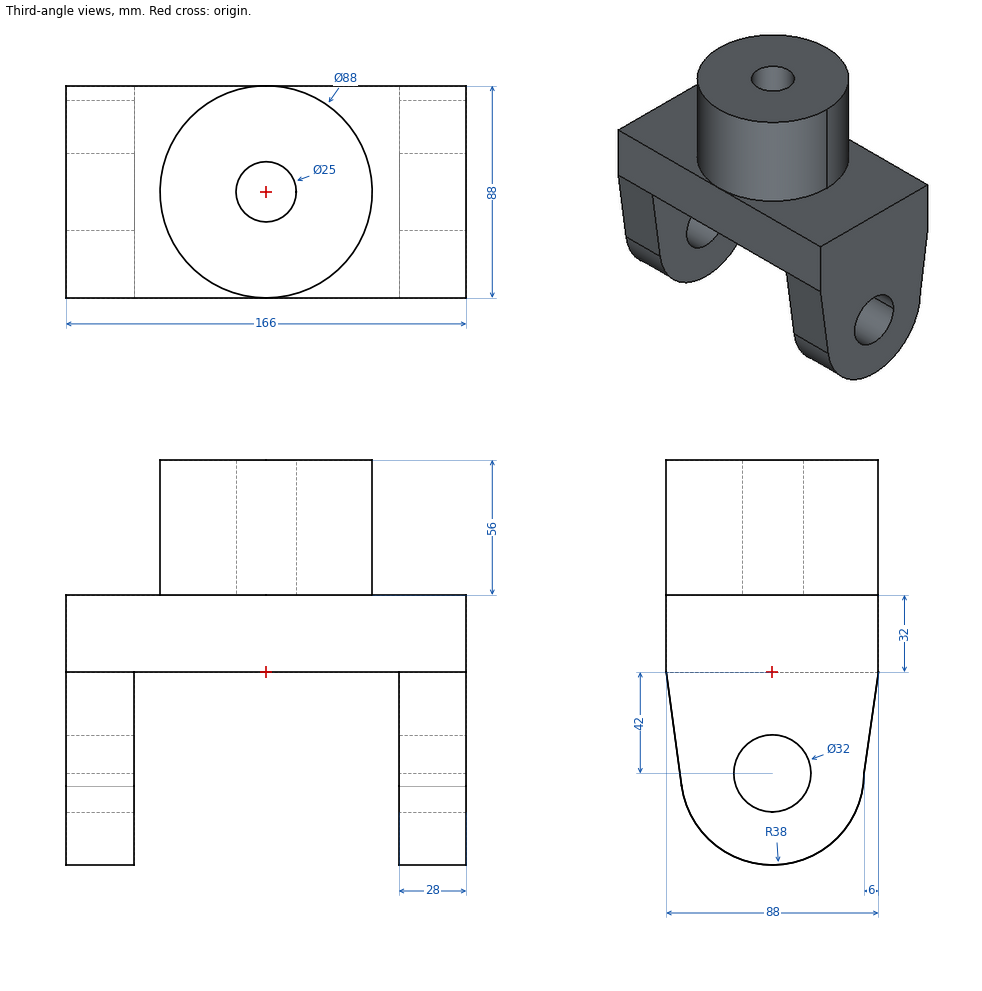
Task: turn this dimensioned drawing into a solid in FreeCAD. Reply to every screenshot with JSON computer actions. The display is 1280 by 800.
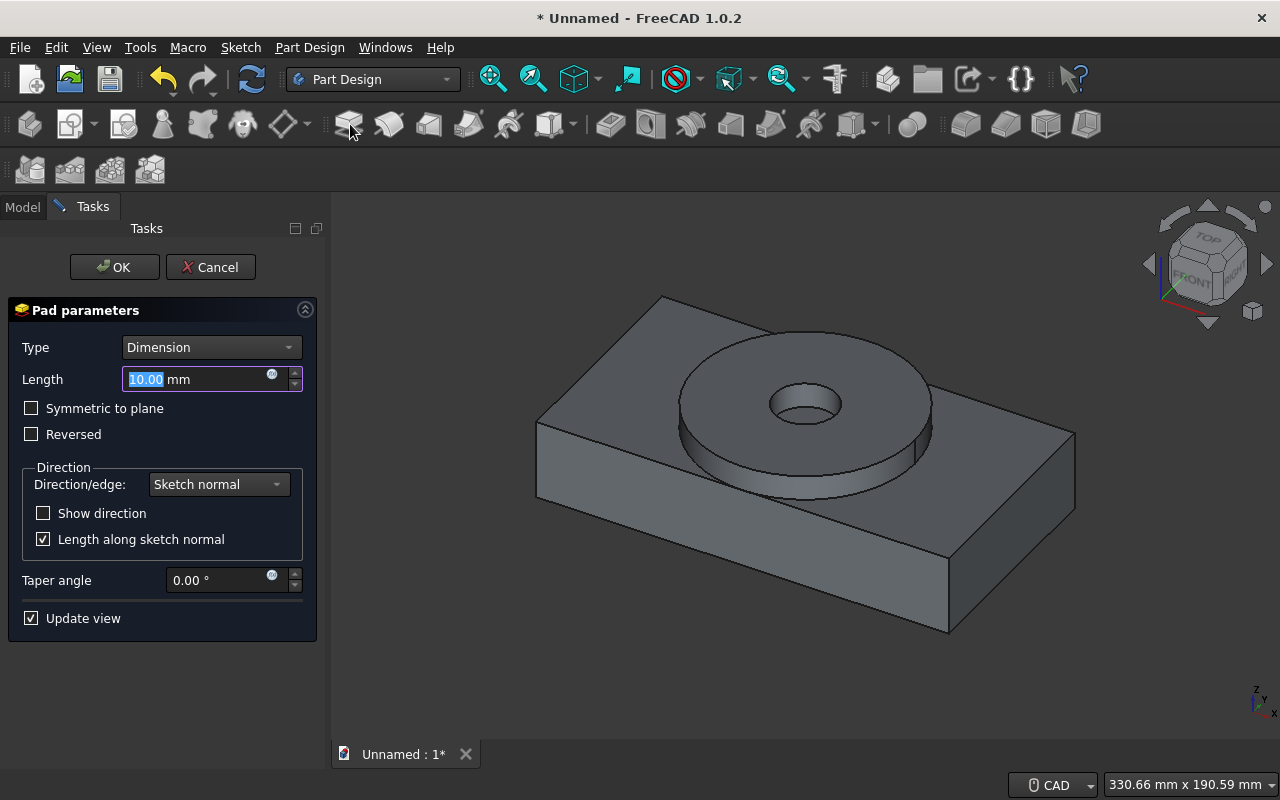
{"action": "type", "text": "56"}
{"action": "key", "text": "Tab"}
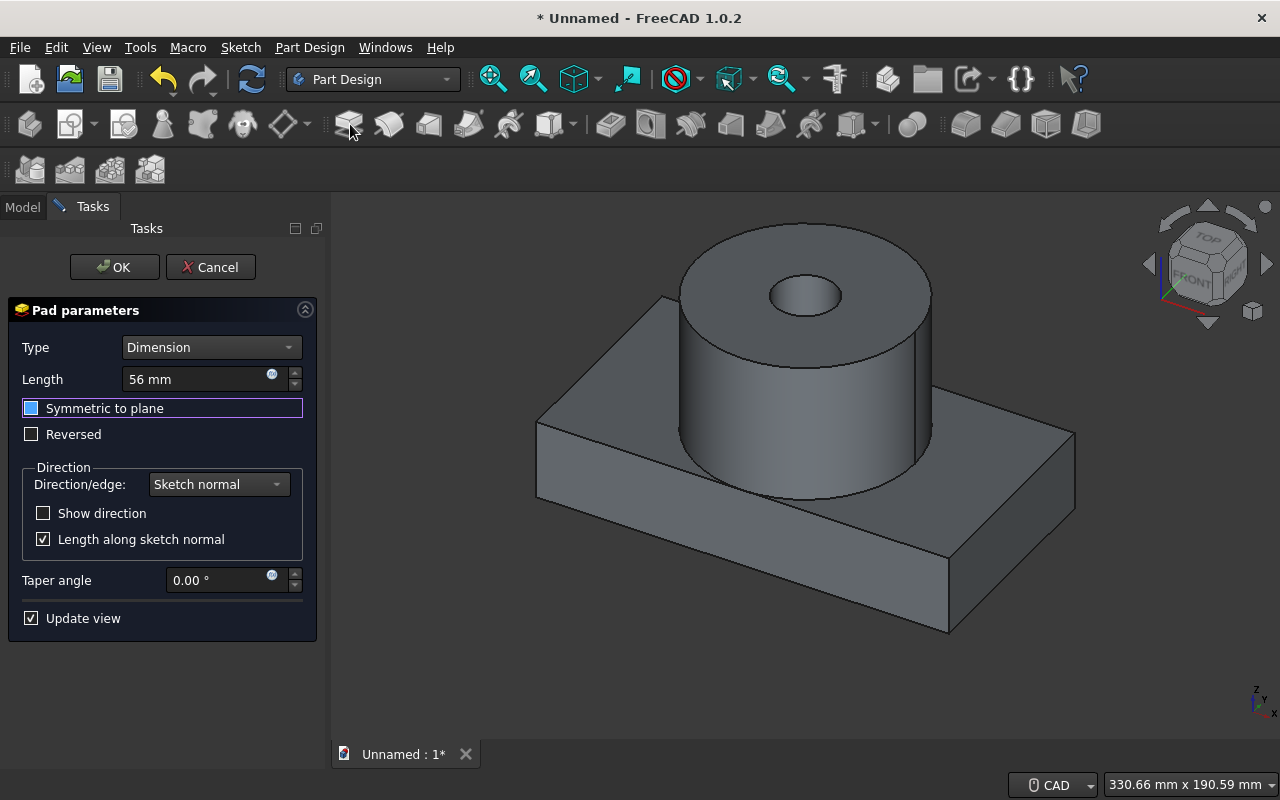
{"action": "left_click", "coordinate": [115, 267]}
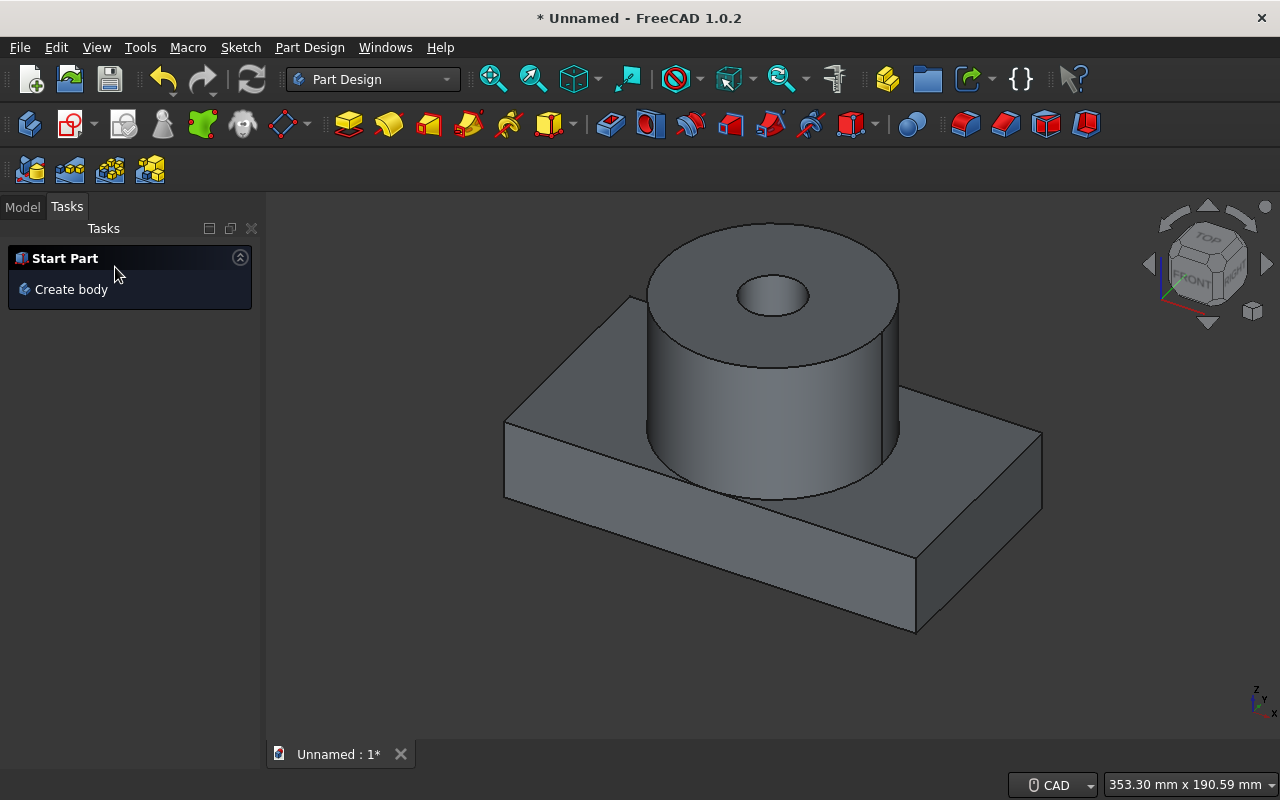
{"action": "left_click", "coordinate": [494, 80]}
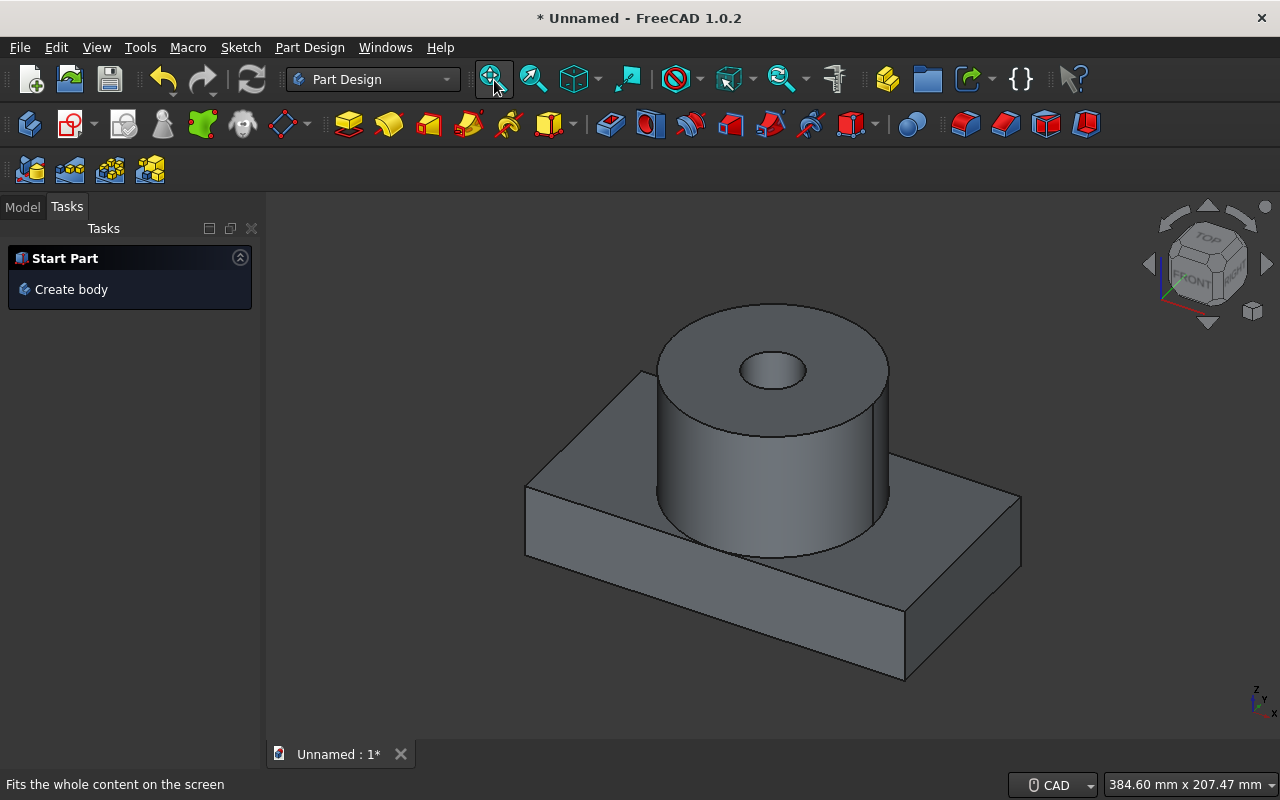
{"action": "left_click", "coordinate": [996, 555]}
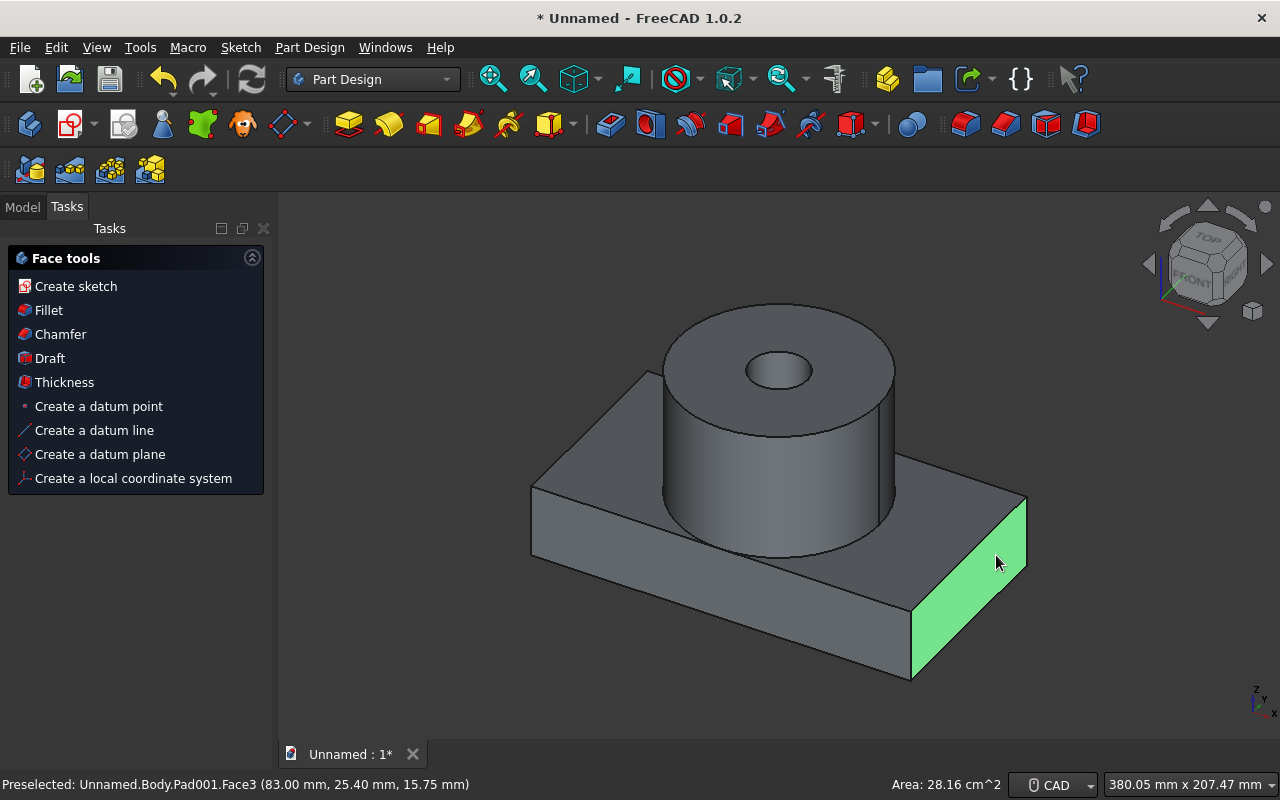
{"action": "left_click", "coordinate": [70, 124]}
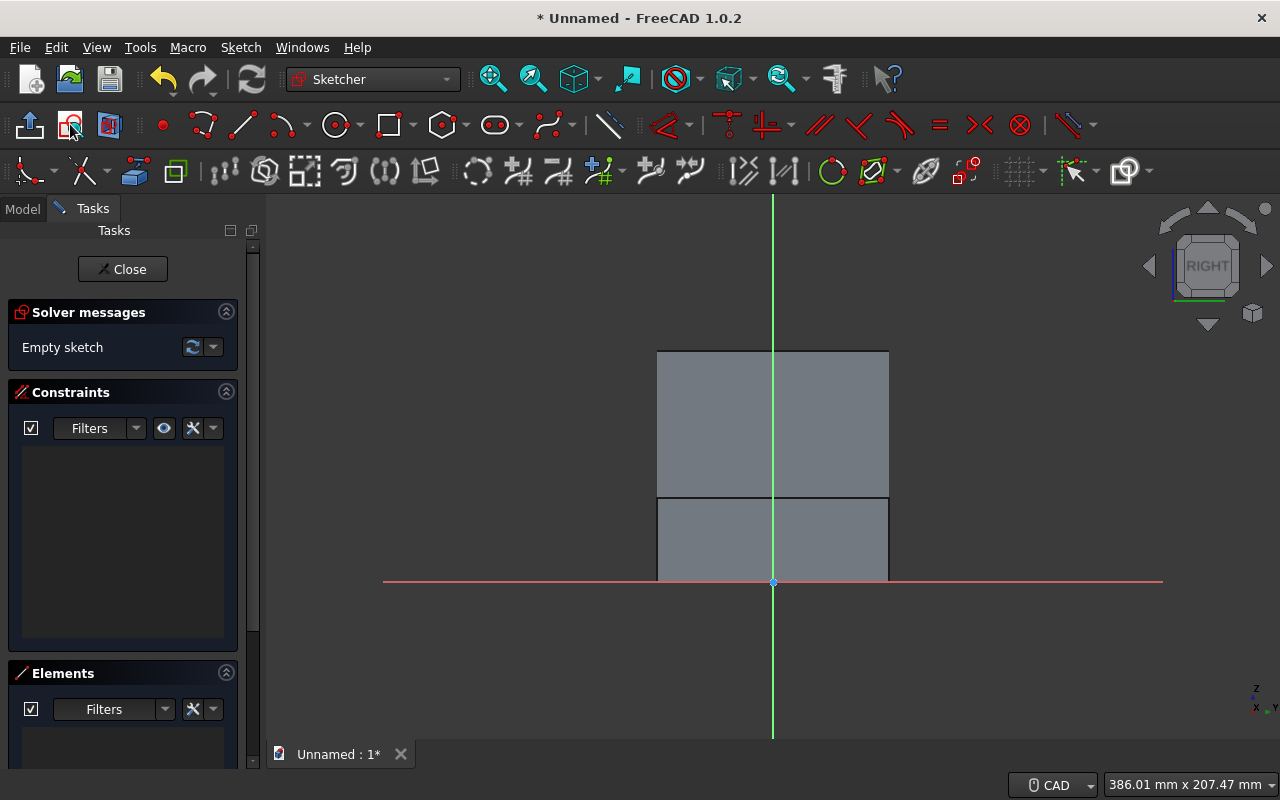
{"action": "scroll", "coordinate": [704, 466], "scroll_direction": "down", "scroll_amount": 5}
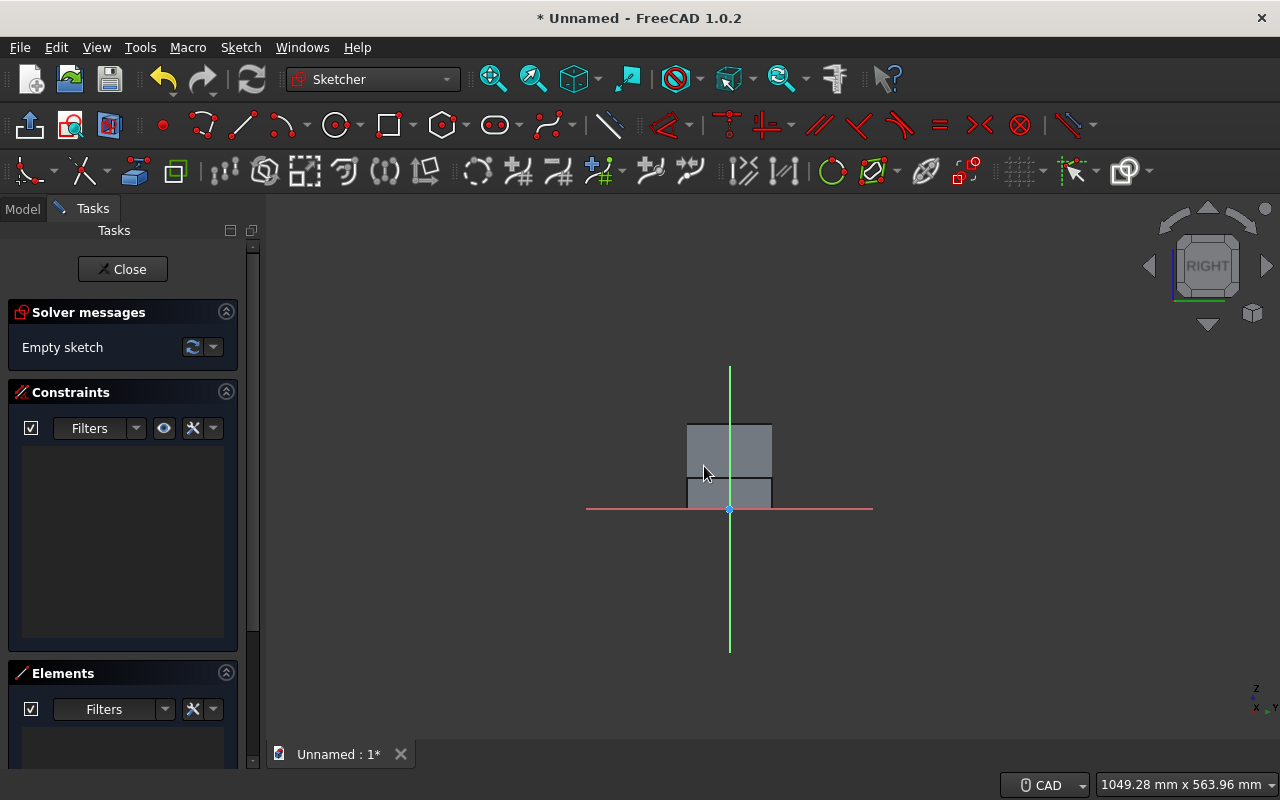
{"action": "scroll", "coordinate": [738, 574], "scroll_direction": "up", "scroll_amount": 7}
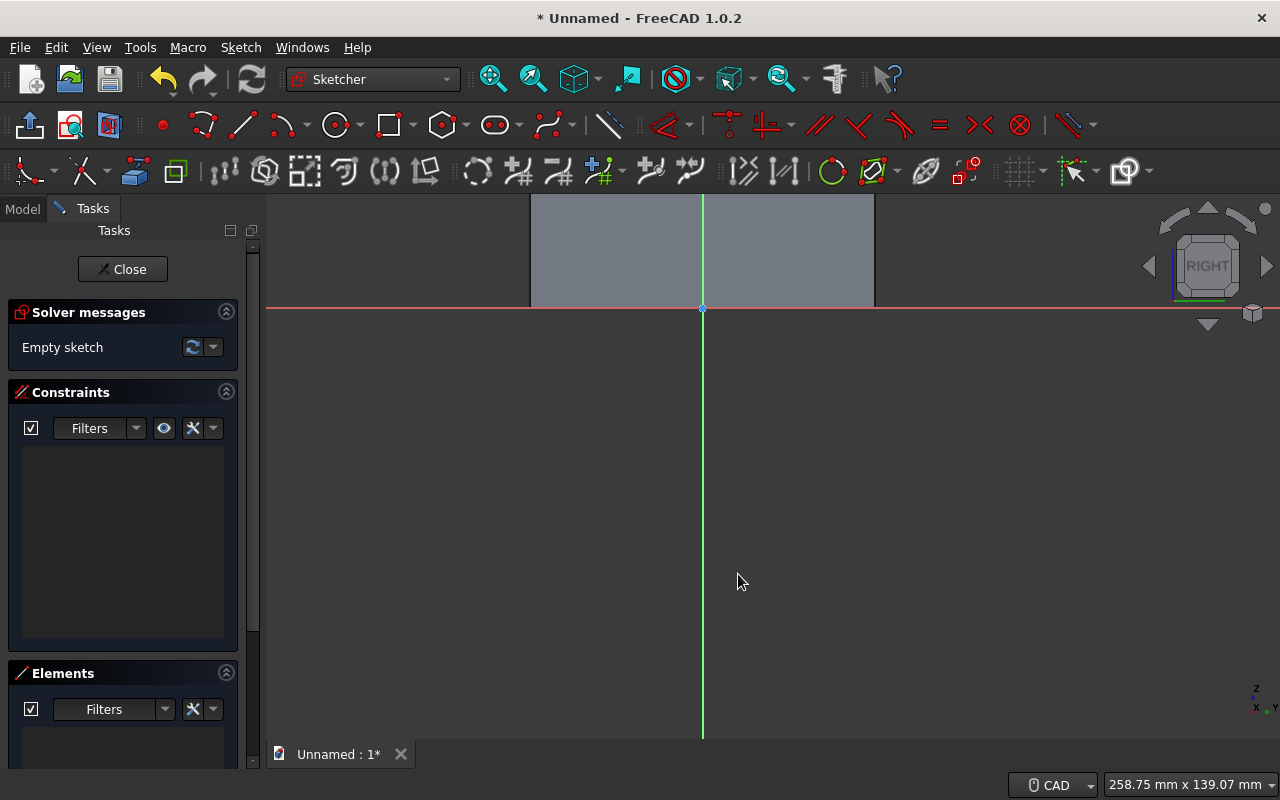
{"action": "left_click", "coordinate": [204, 126]}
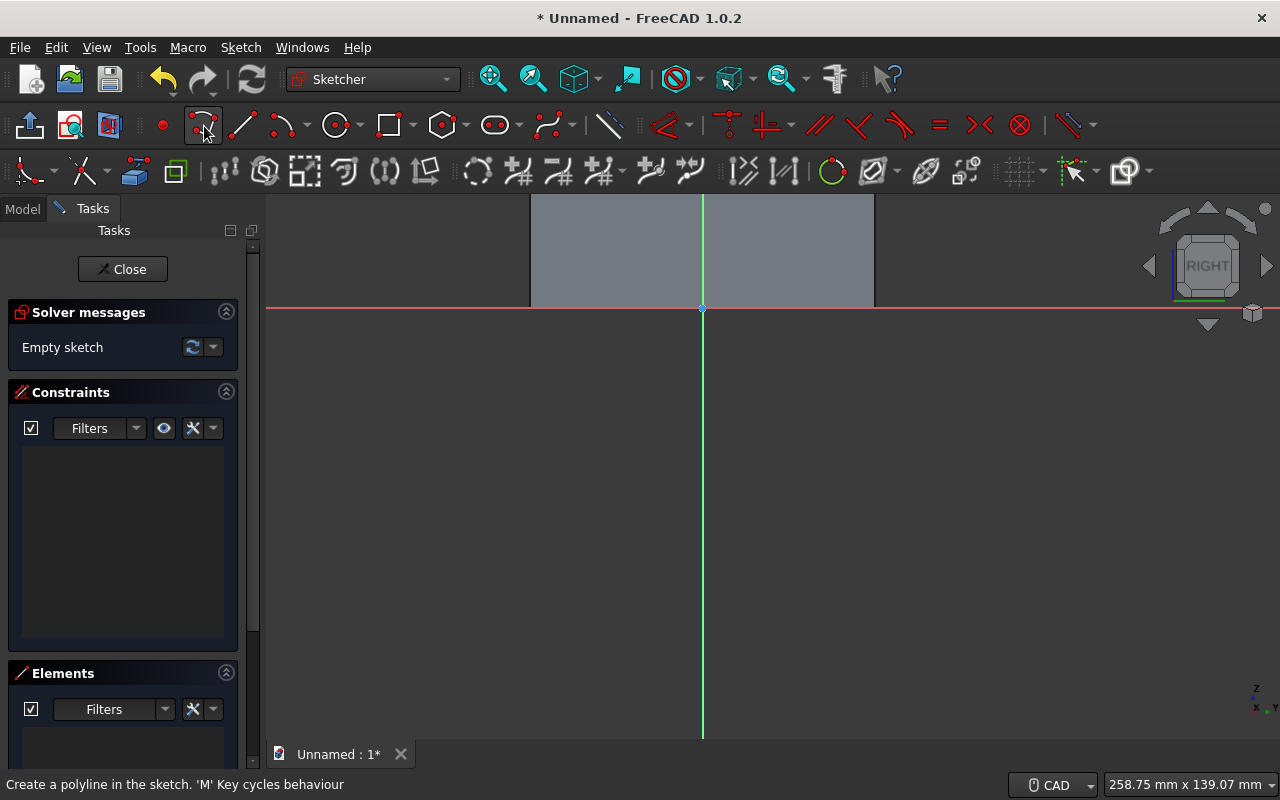
{"action": "left_click", "coordinate": [852, 473]}
{"action": "left_click", "coordinate": [875, 308]}
{"action": "left_click", "coordinate": [530, 317]}
{"action": "left_click", "coordinate": [555, 493]}
{"action": "right_click", "coordinate": [555, 493]}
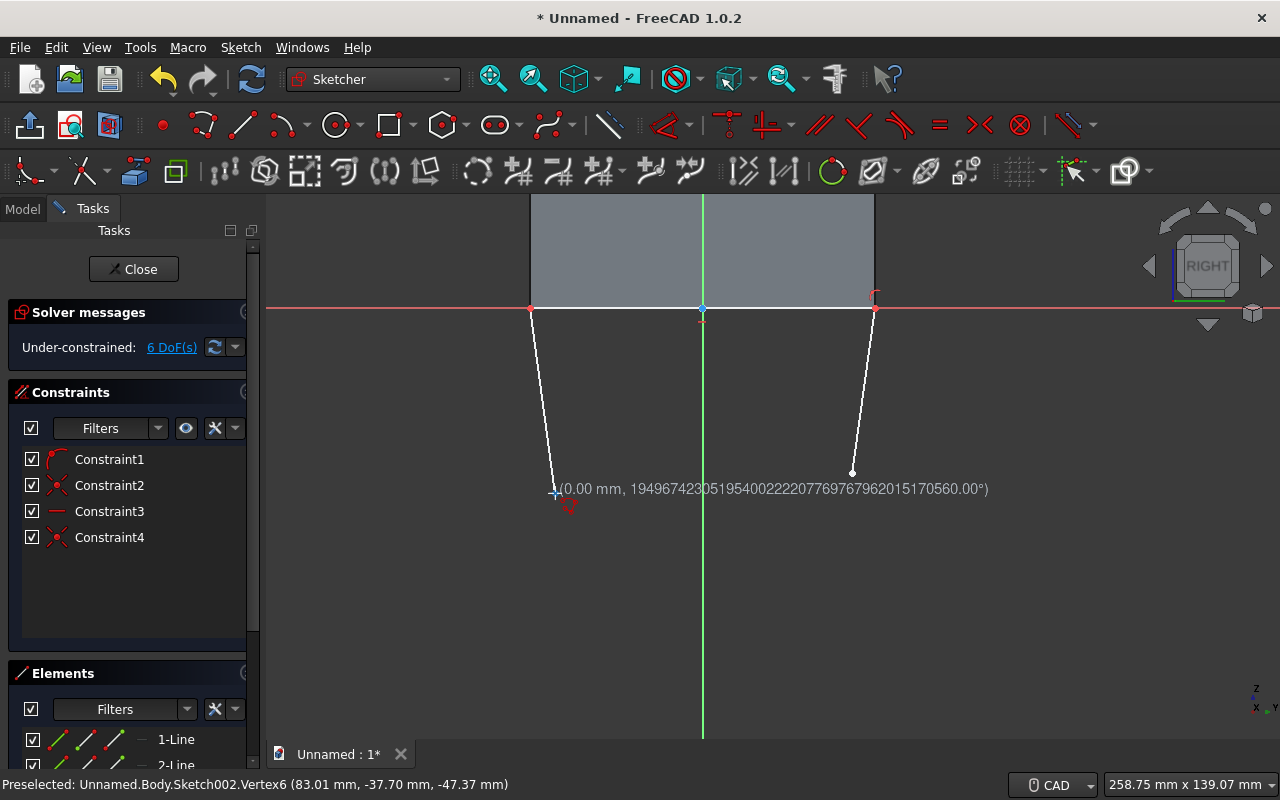
{"action": "left_click", "coordinate": [310, 126]}